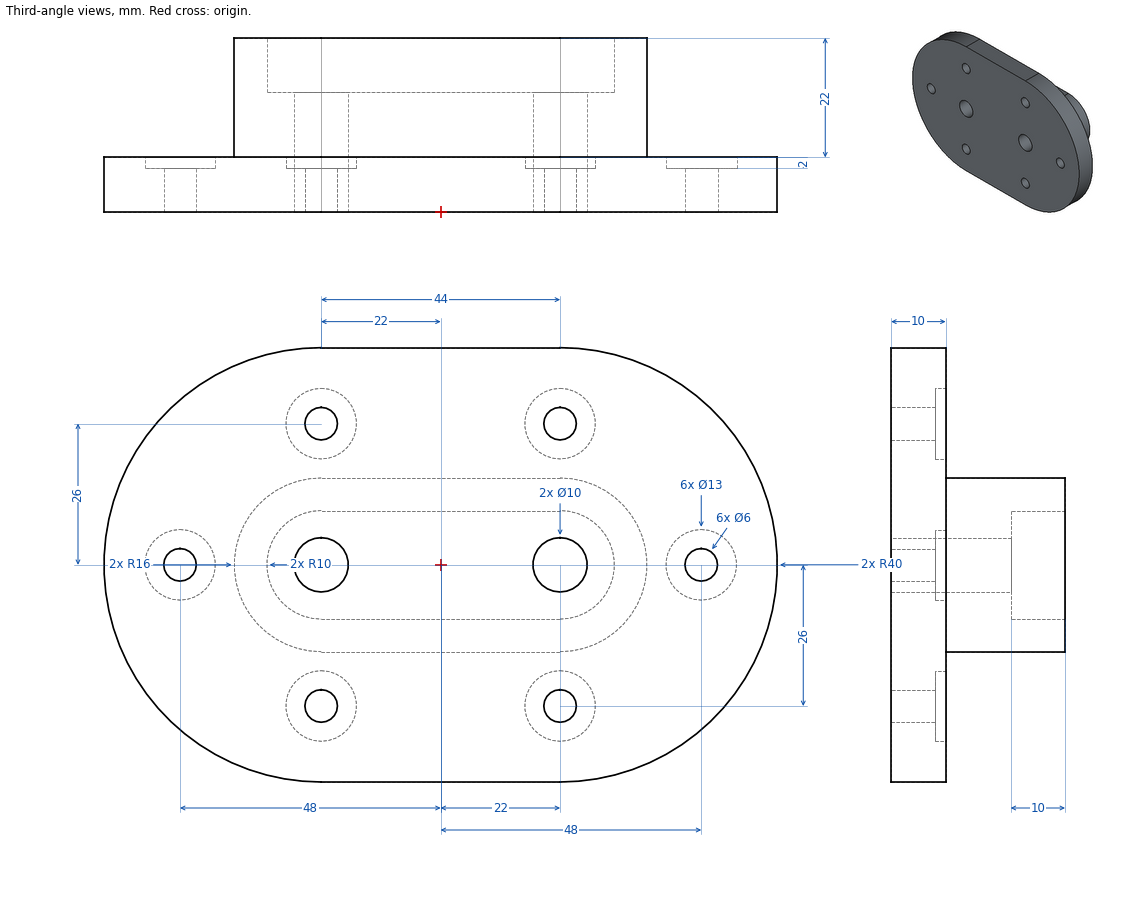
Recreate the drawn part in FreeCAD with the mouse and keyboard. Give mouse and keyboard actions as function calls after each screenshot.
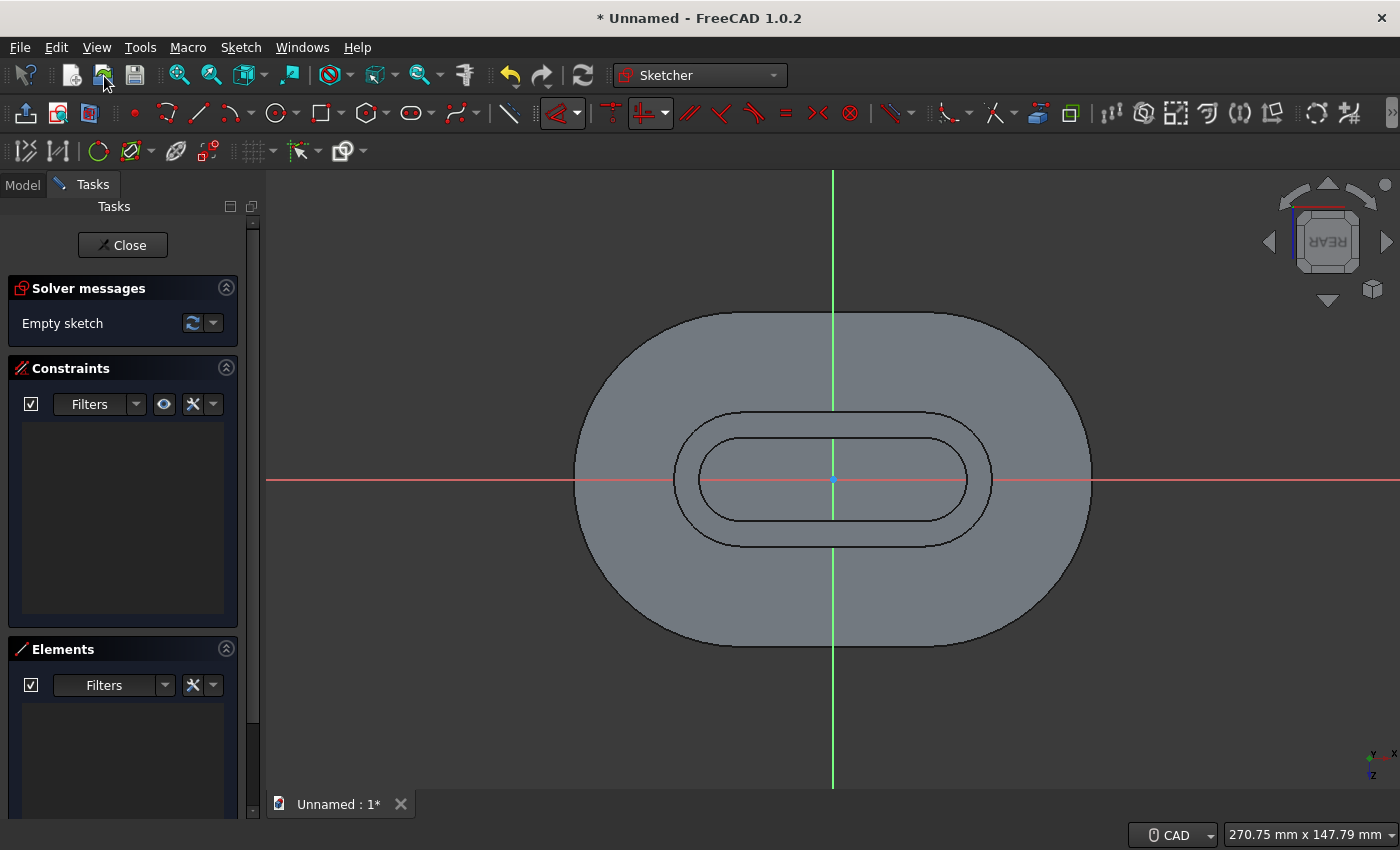
click(90, 114)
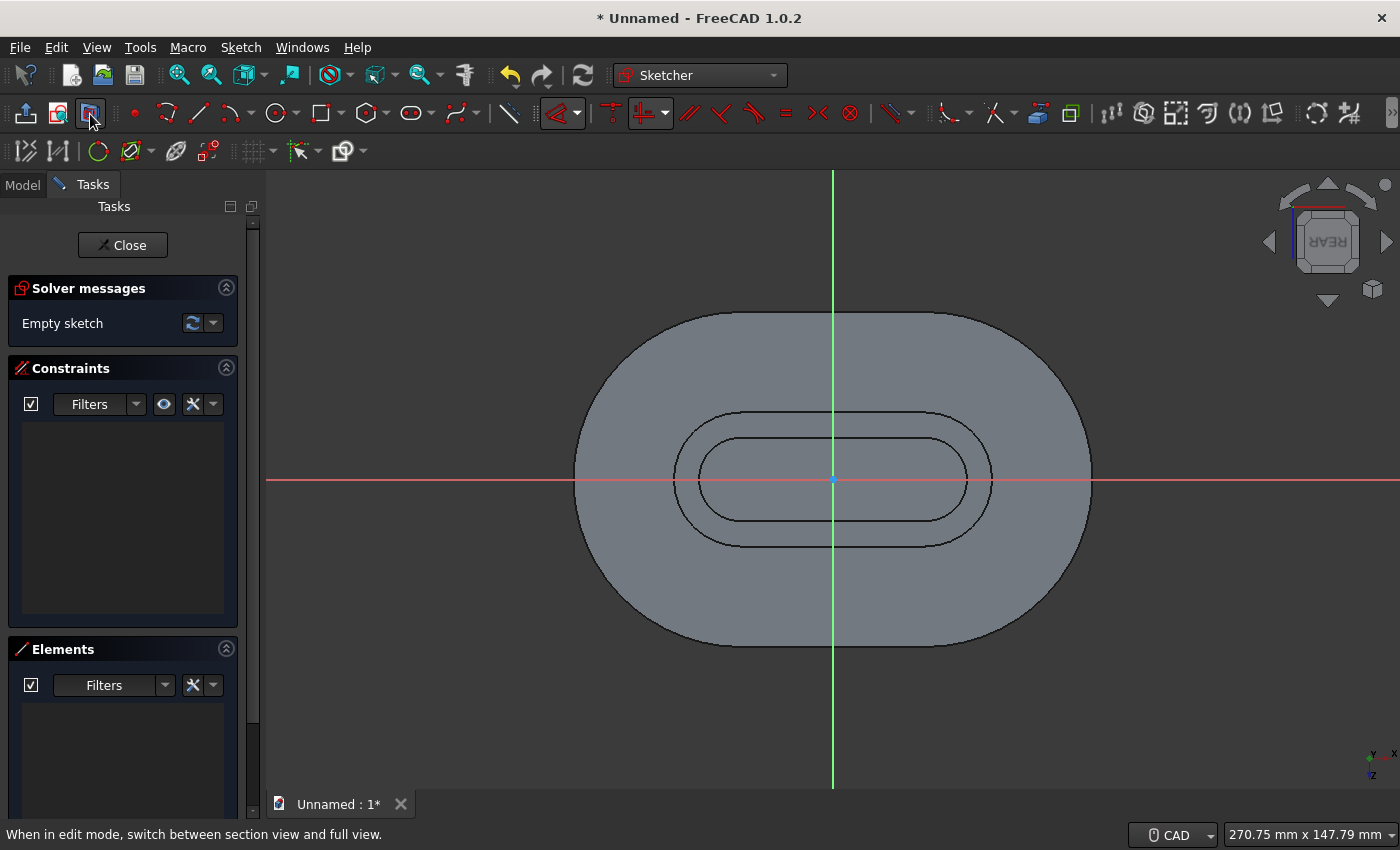
scroll(873, 479, up, 5)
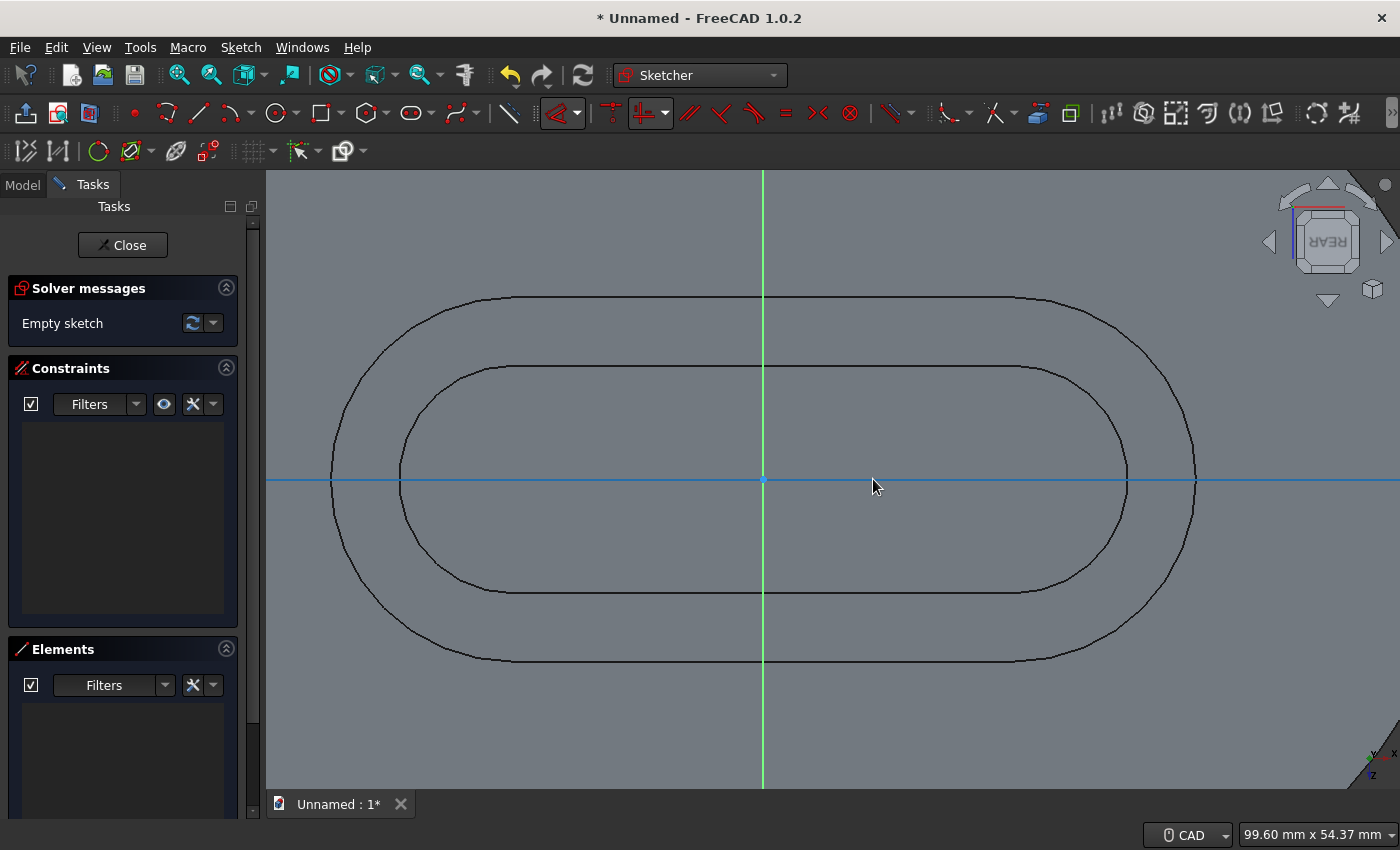
click(276, 114)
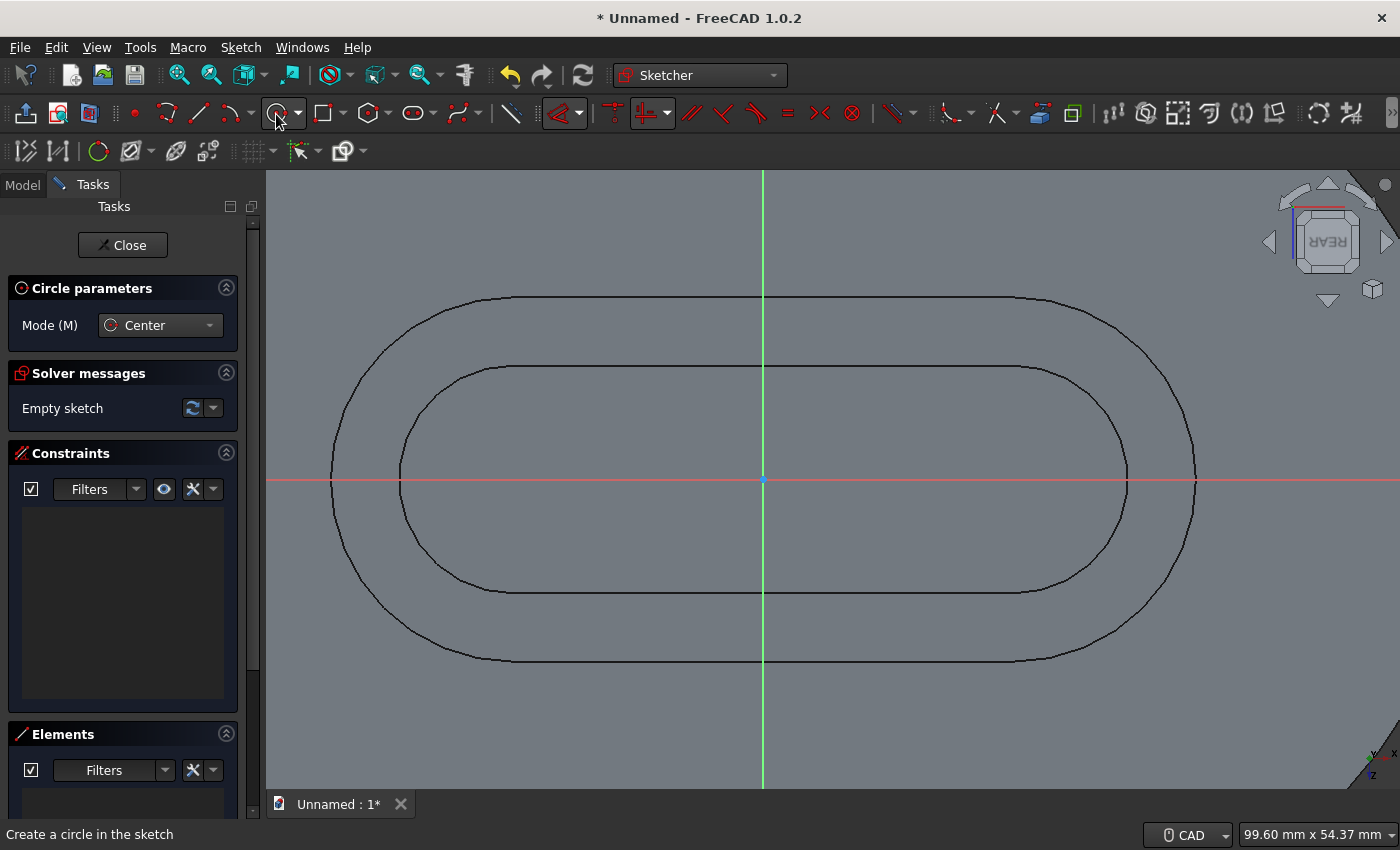
click(1014, 479)
click(1054, 439)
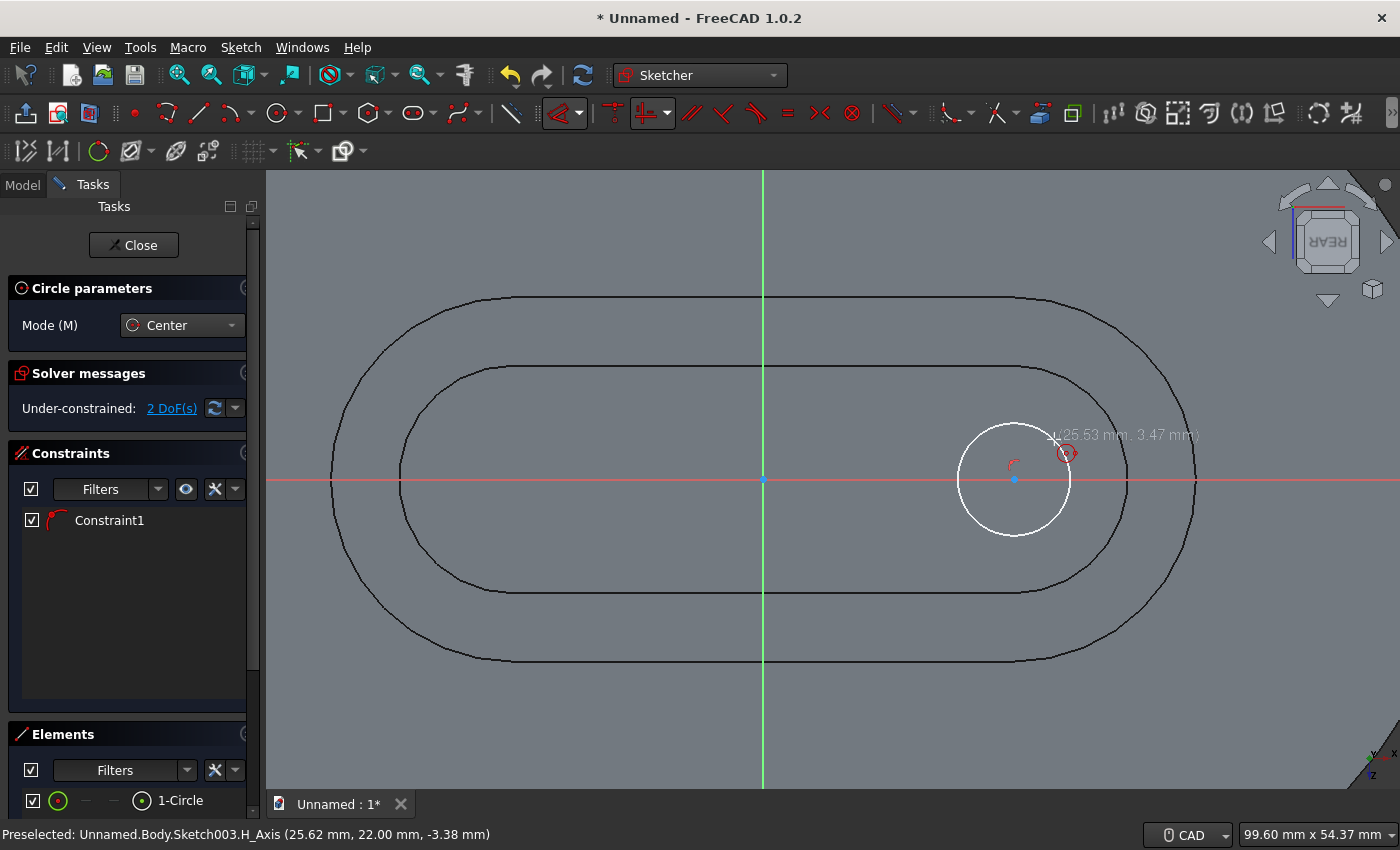
click(513, 479)
click(553, 439)
key(Escape)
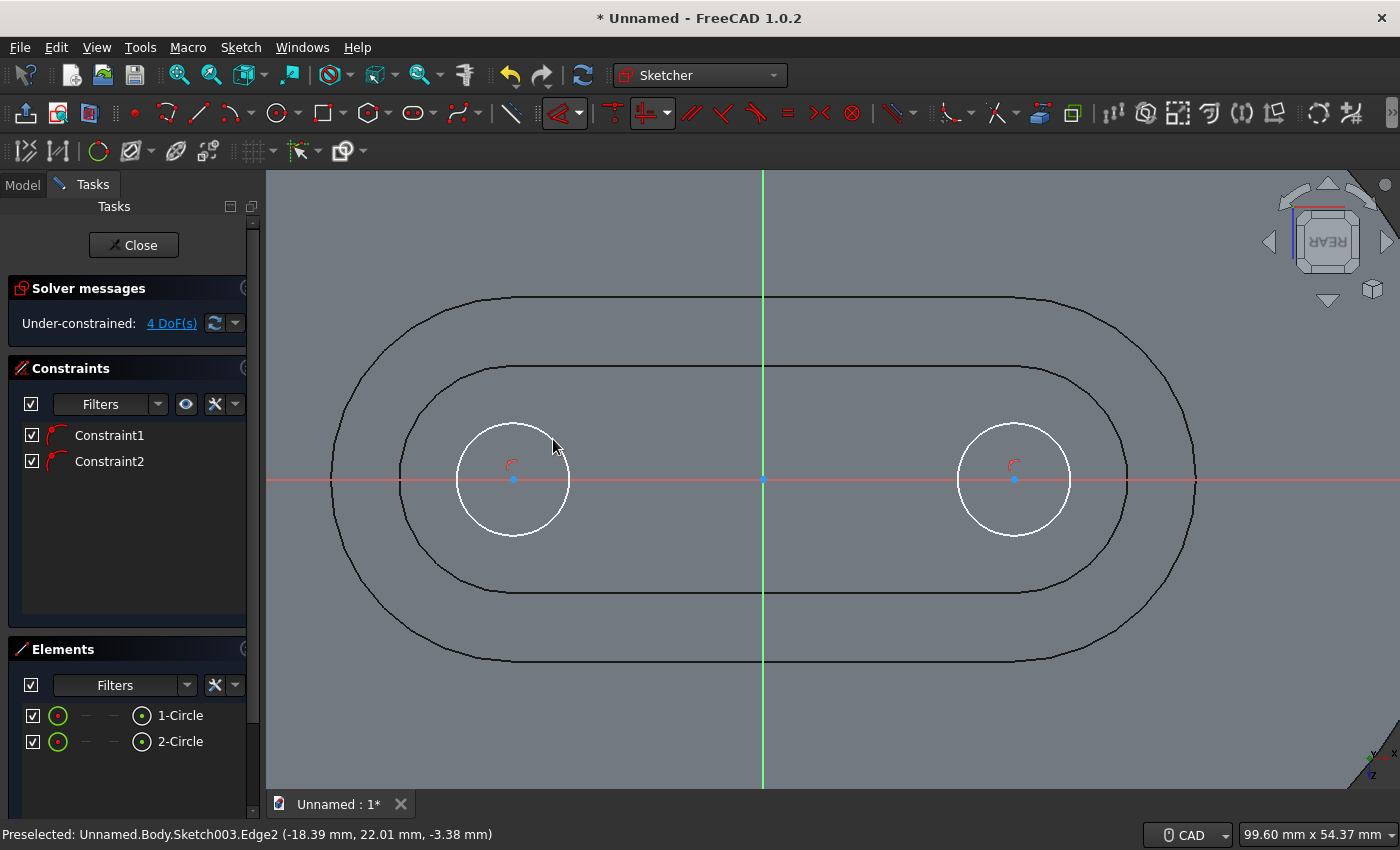
click(1054, 440)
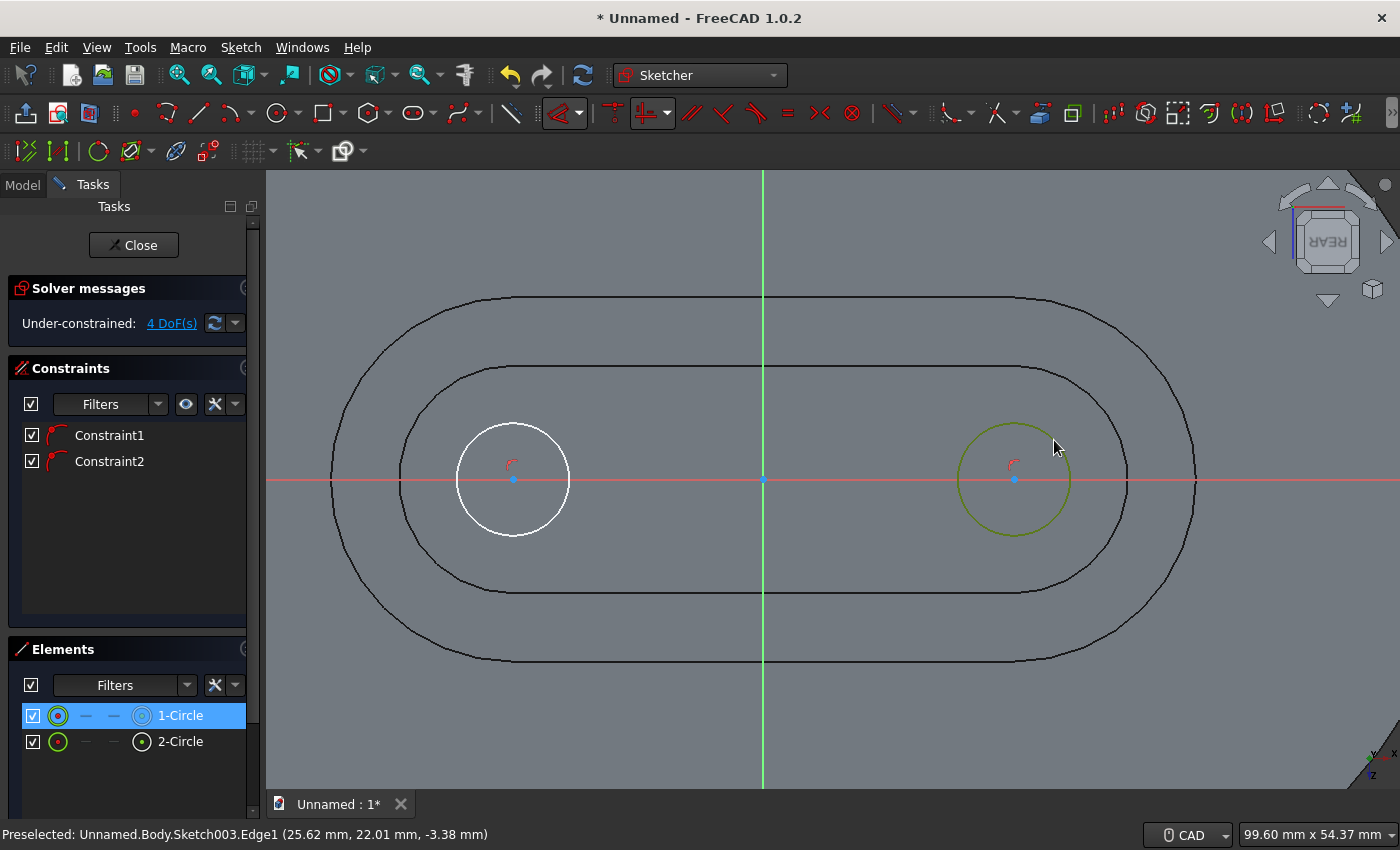
click(553, 440)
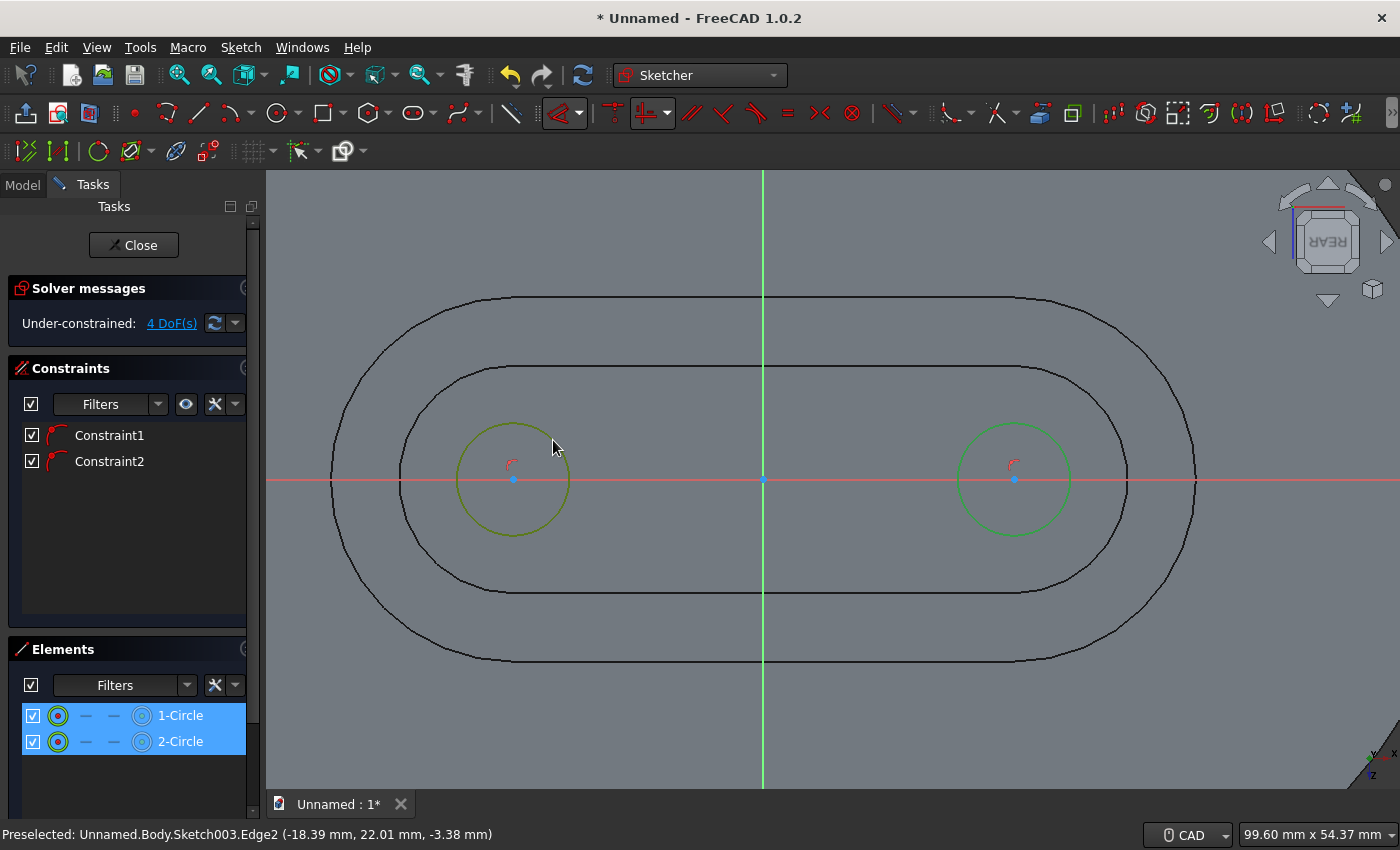
key(e)